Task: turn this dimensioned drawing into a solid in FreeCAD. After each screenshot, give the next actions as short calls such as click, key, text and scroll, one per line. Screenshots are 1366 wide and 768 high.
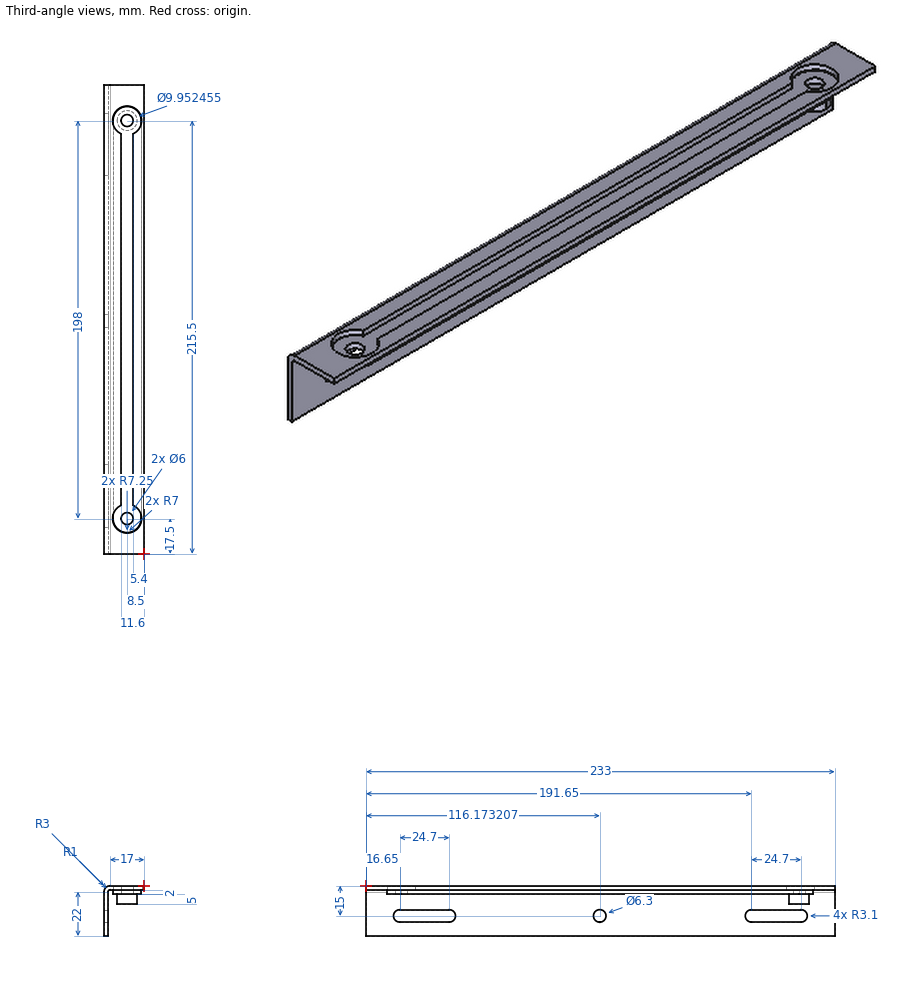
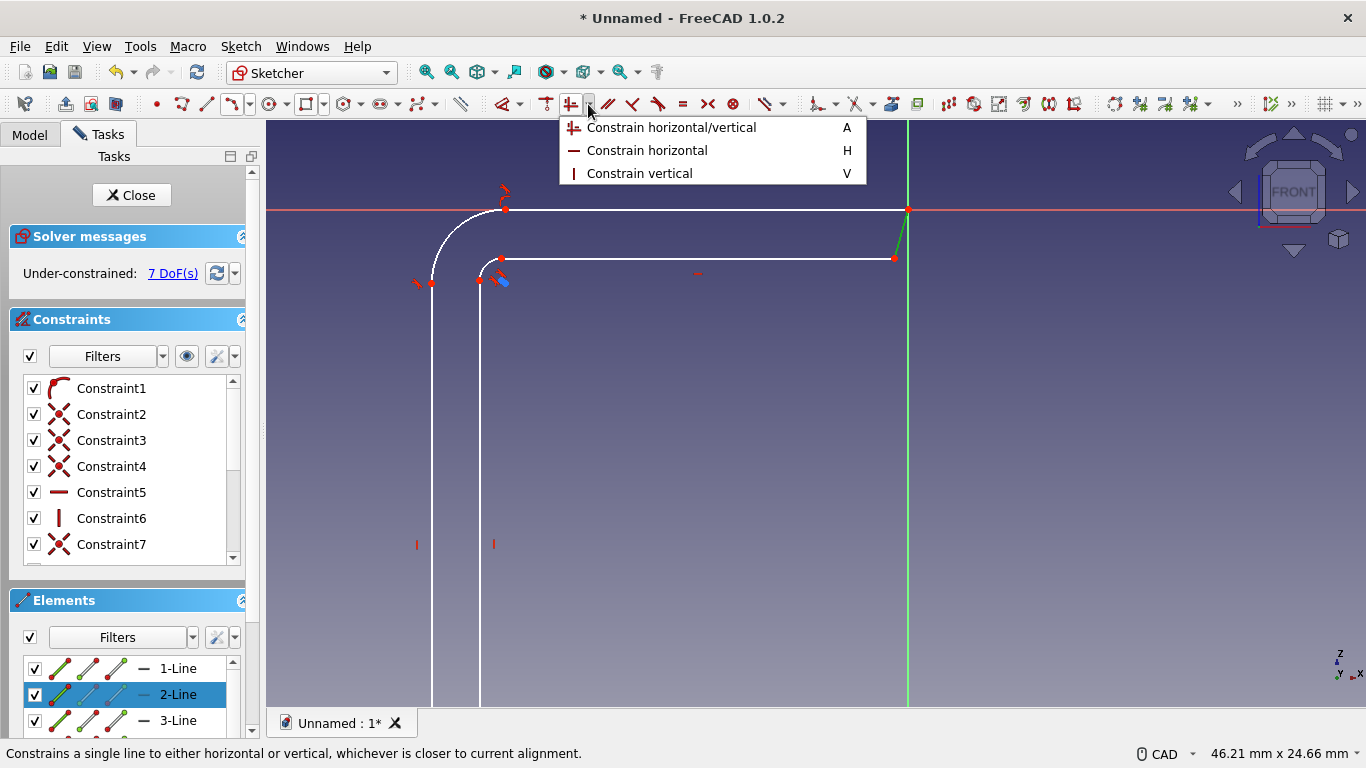
click(713, 174)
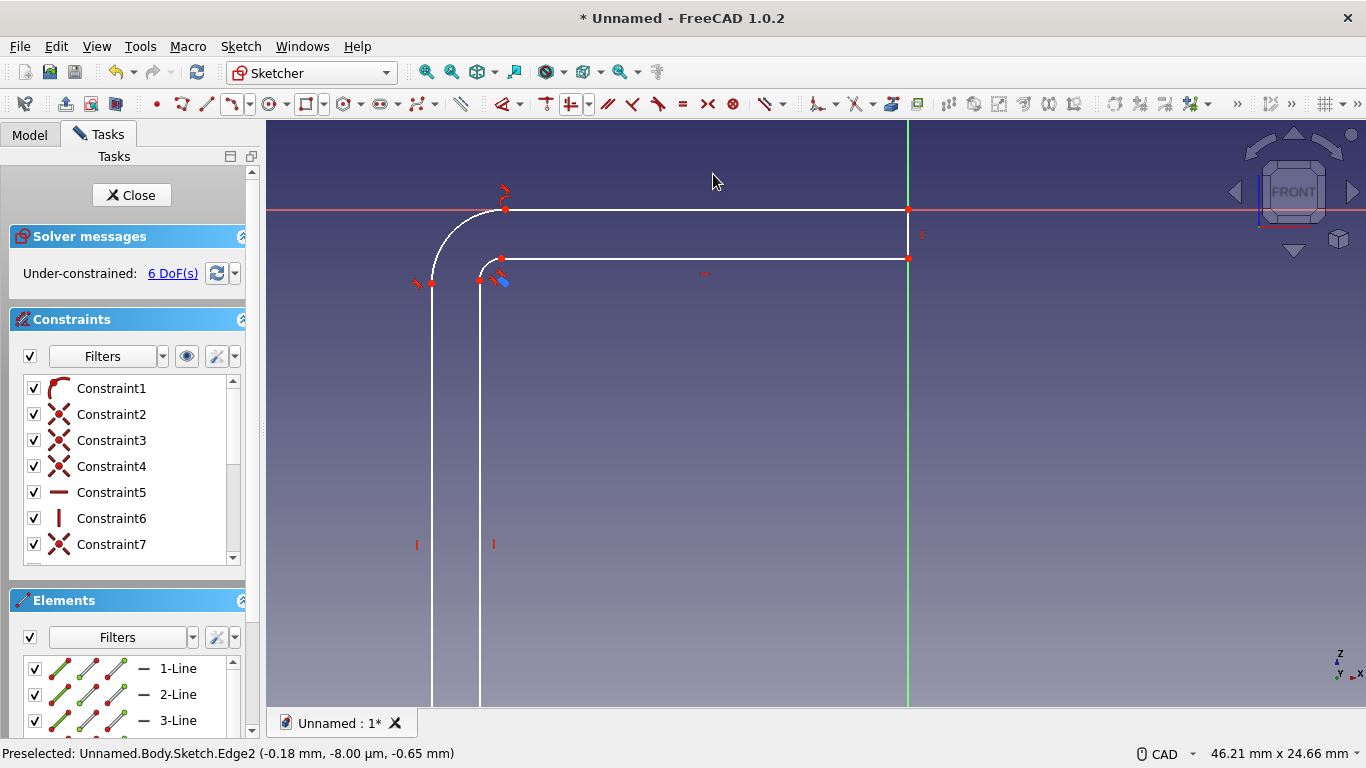
scroll(492, 261, up, 2)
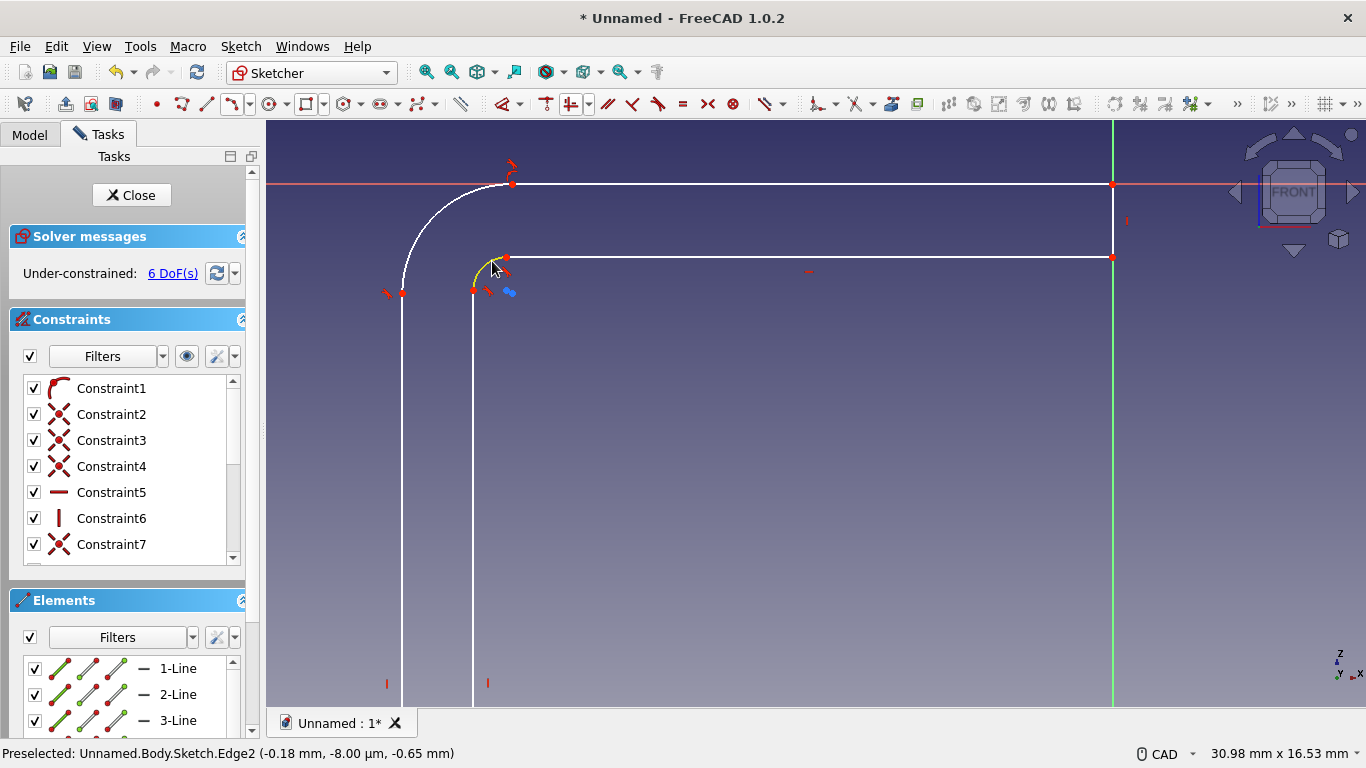
click(492, 261)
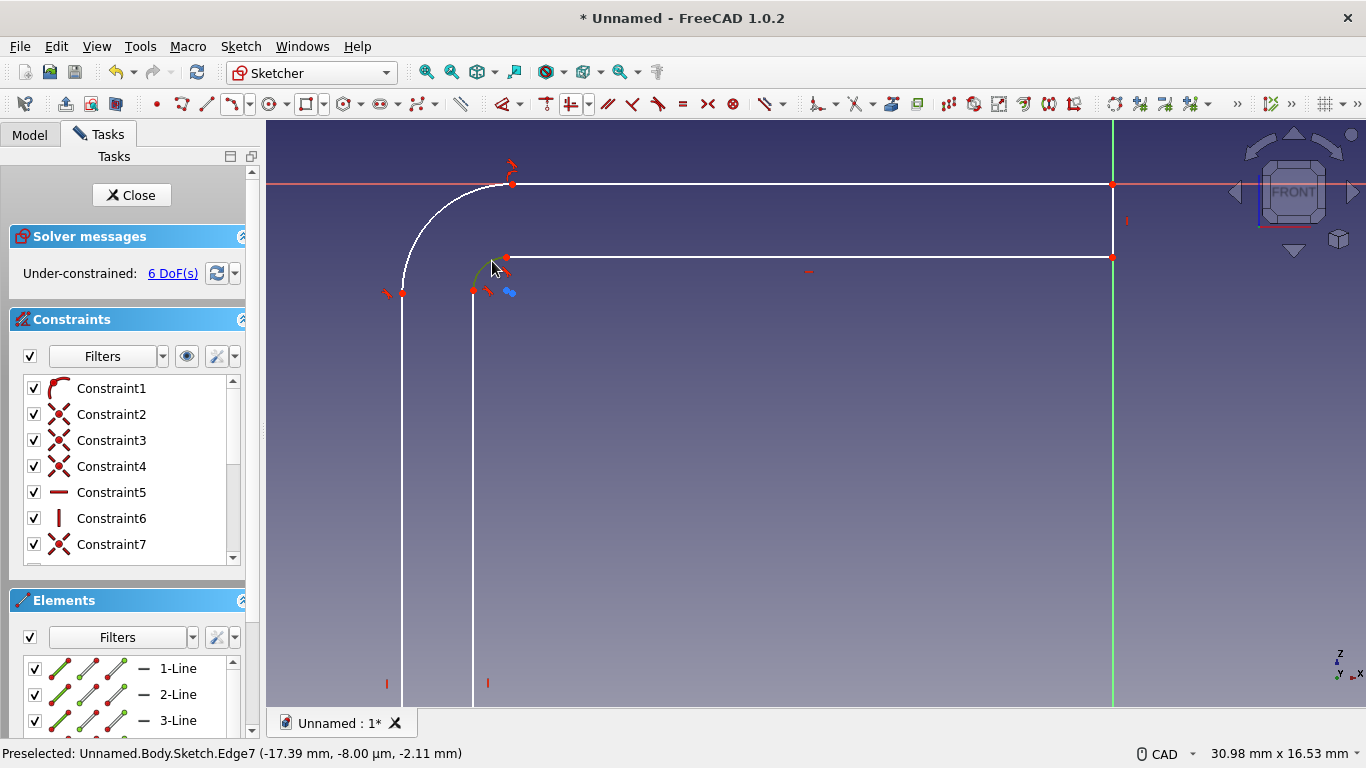
click(462, 196)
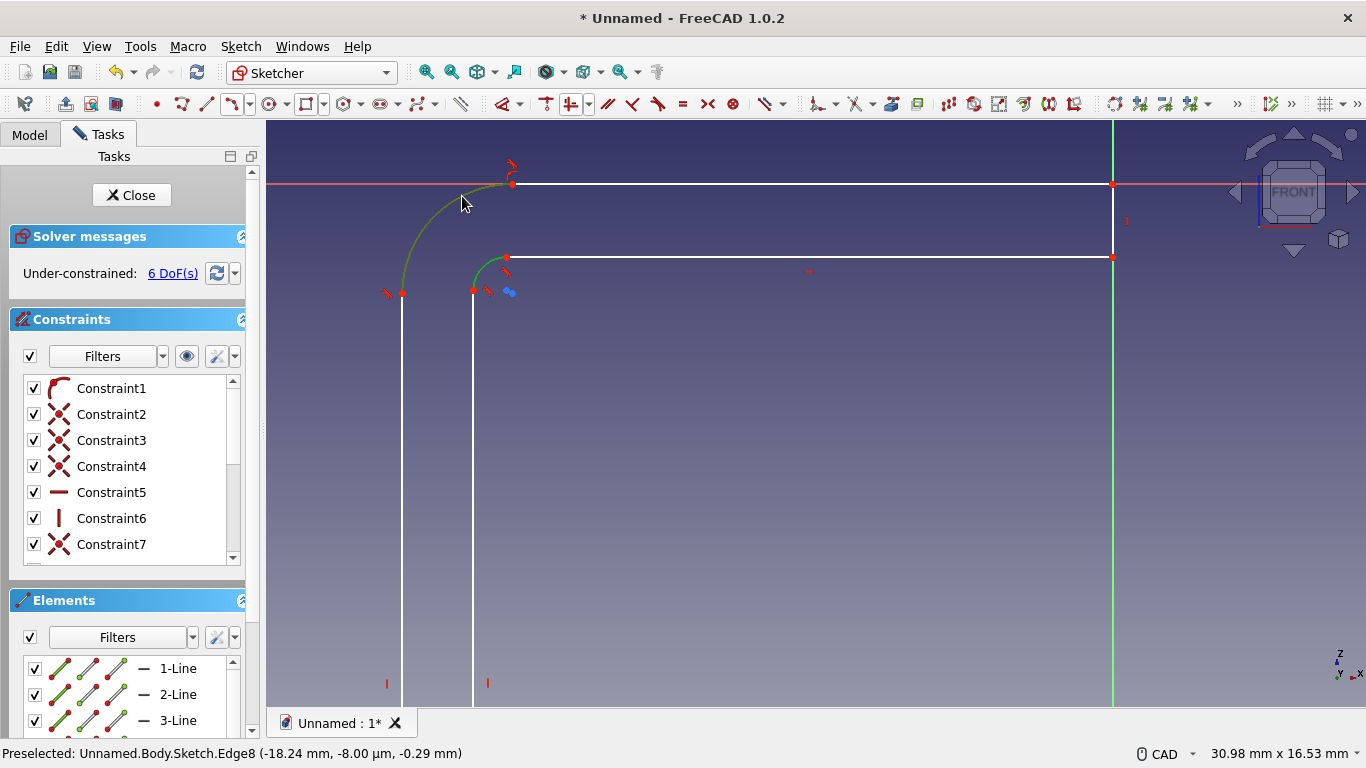
click(546, 104)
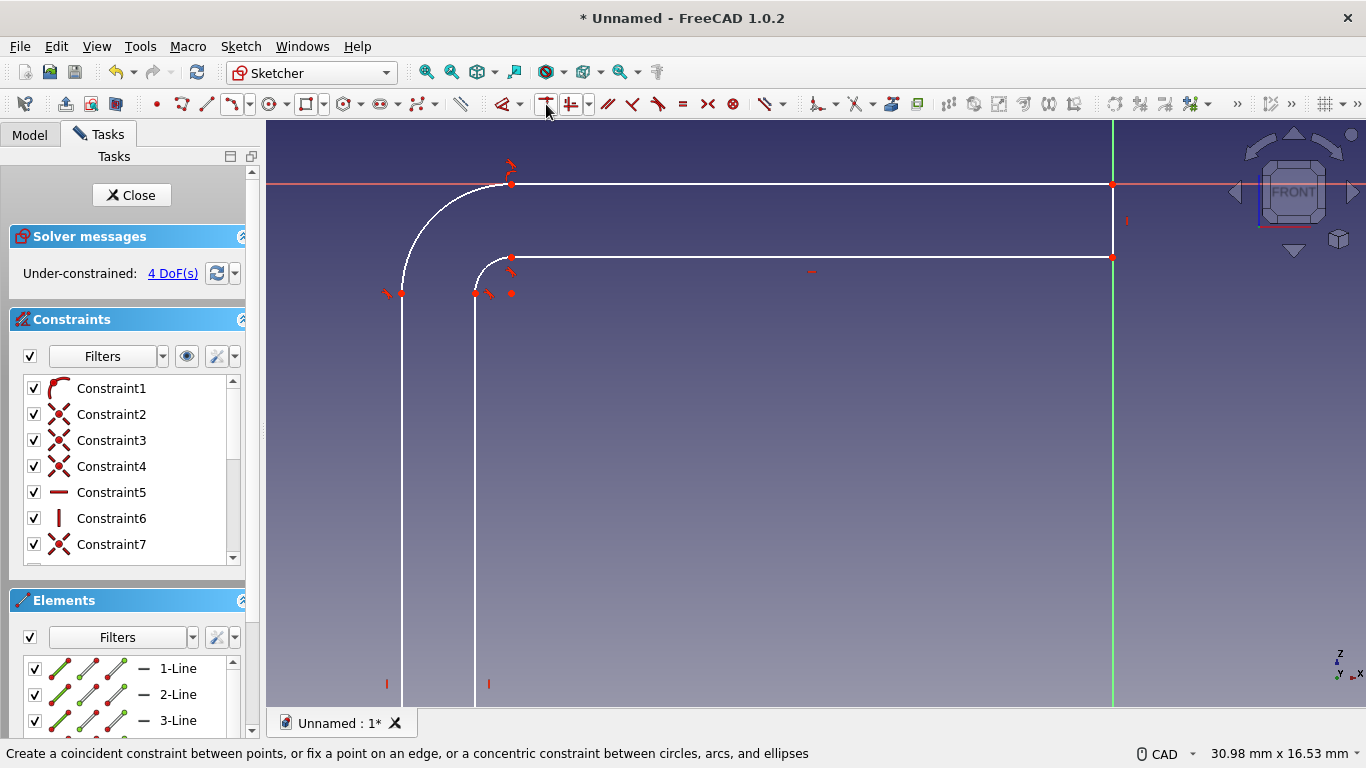
click(495, 261)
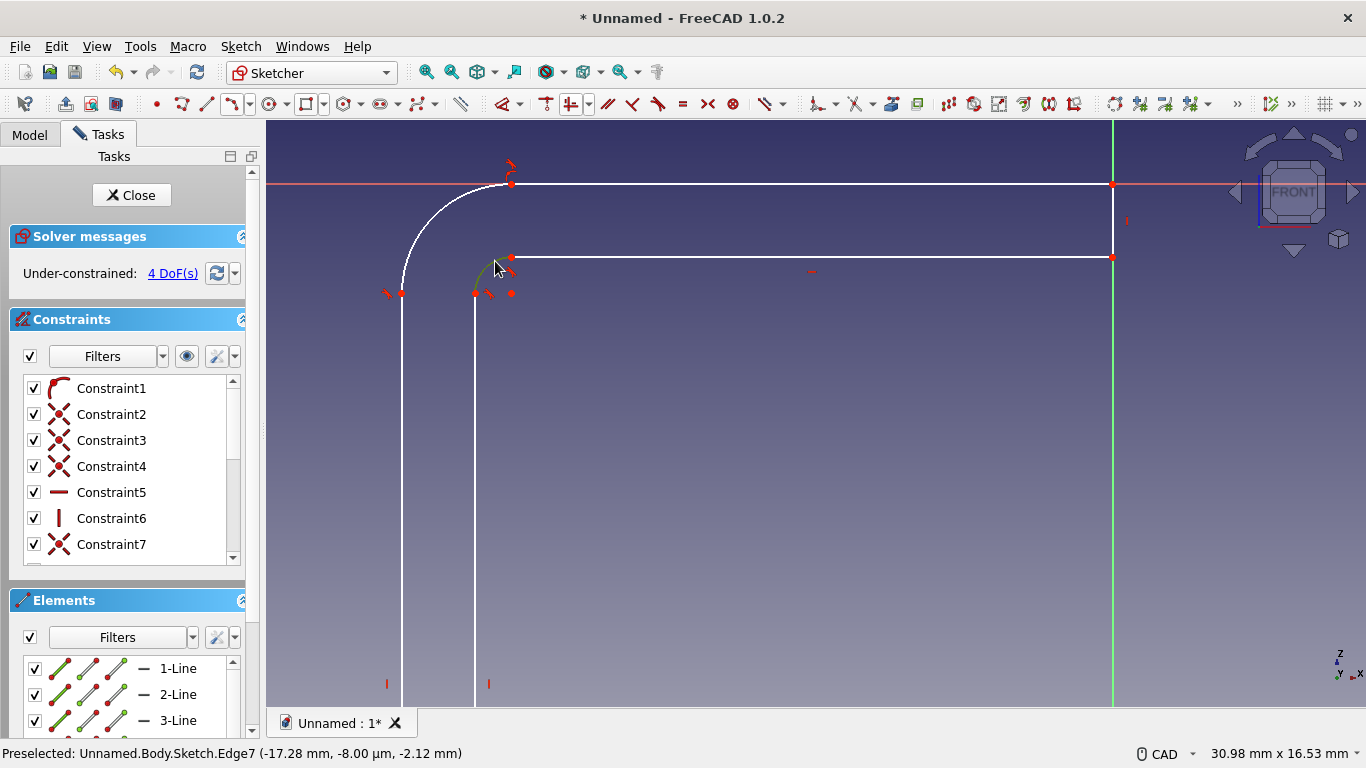
key(k)
key(r)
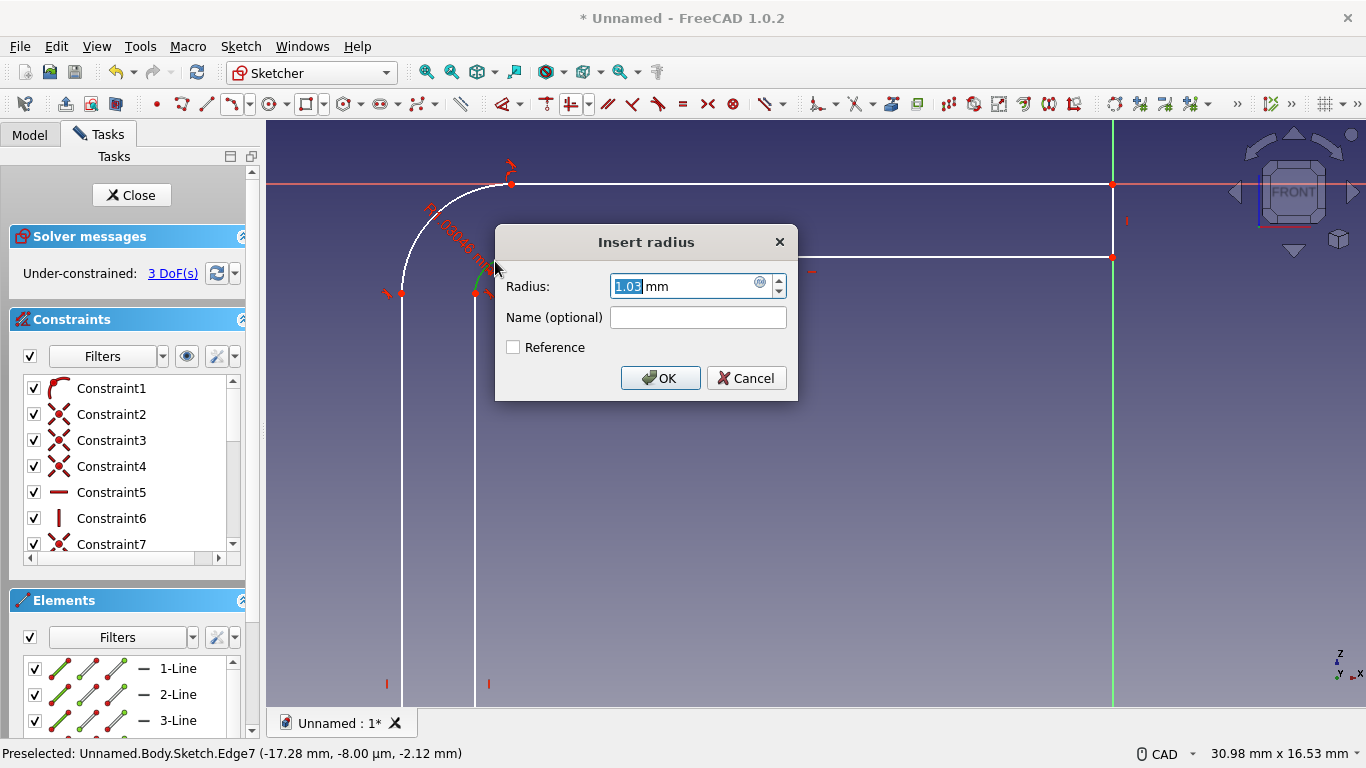
text(1)
key(Return)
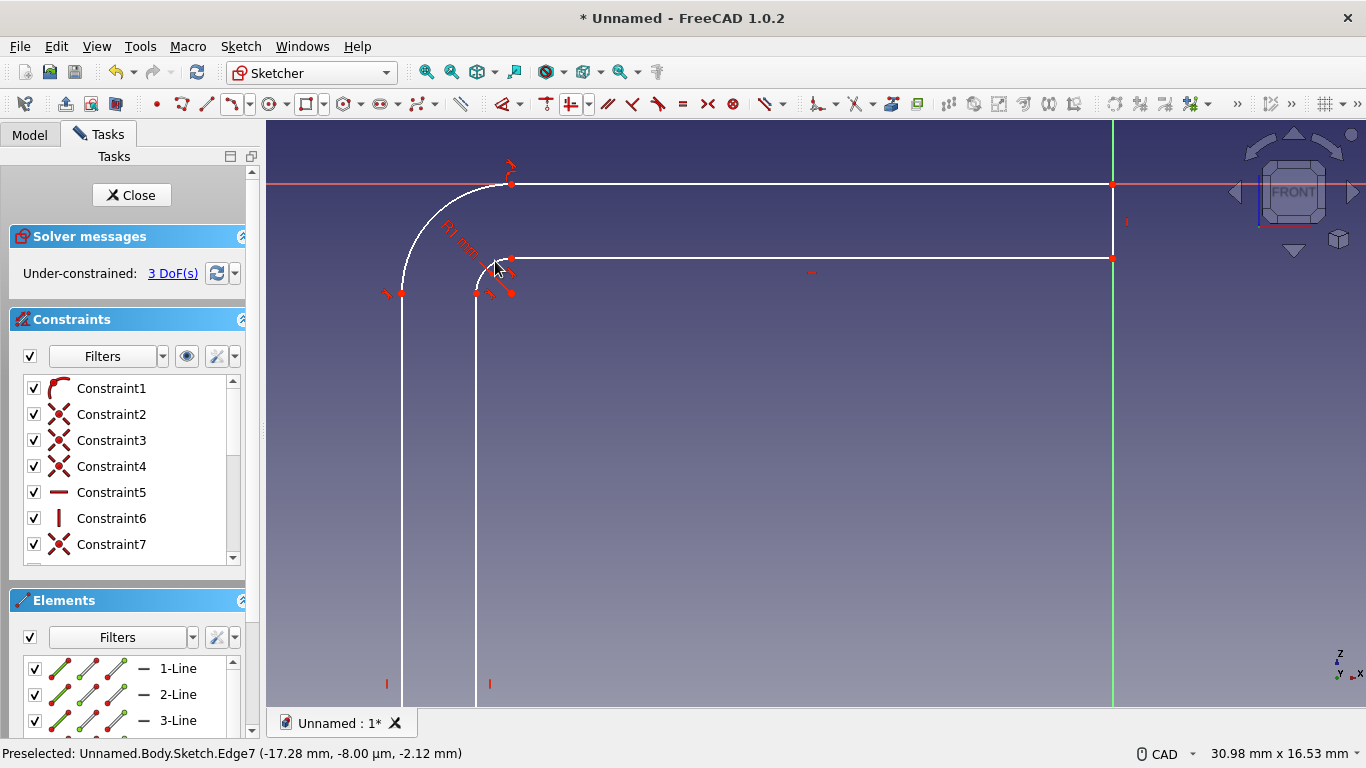
click(462, 196)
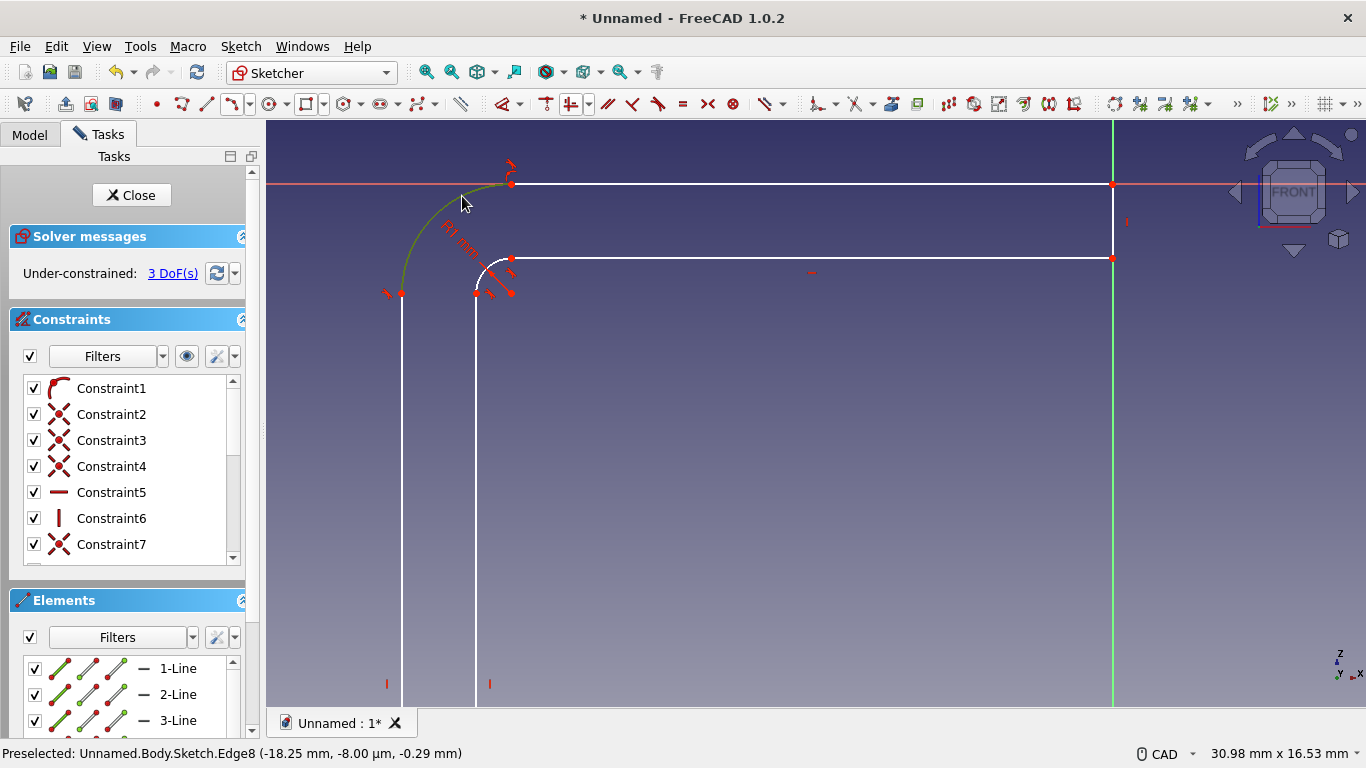
key(k)
key(r)